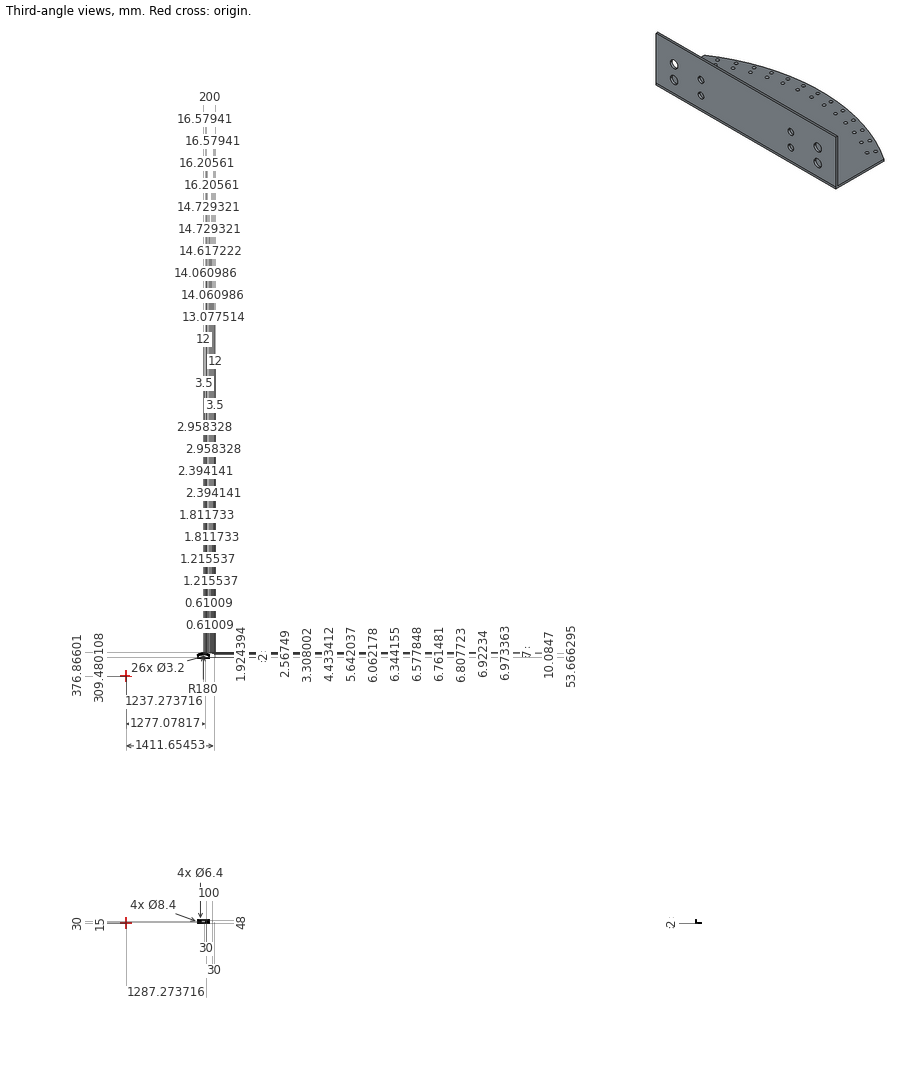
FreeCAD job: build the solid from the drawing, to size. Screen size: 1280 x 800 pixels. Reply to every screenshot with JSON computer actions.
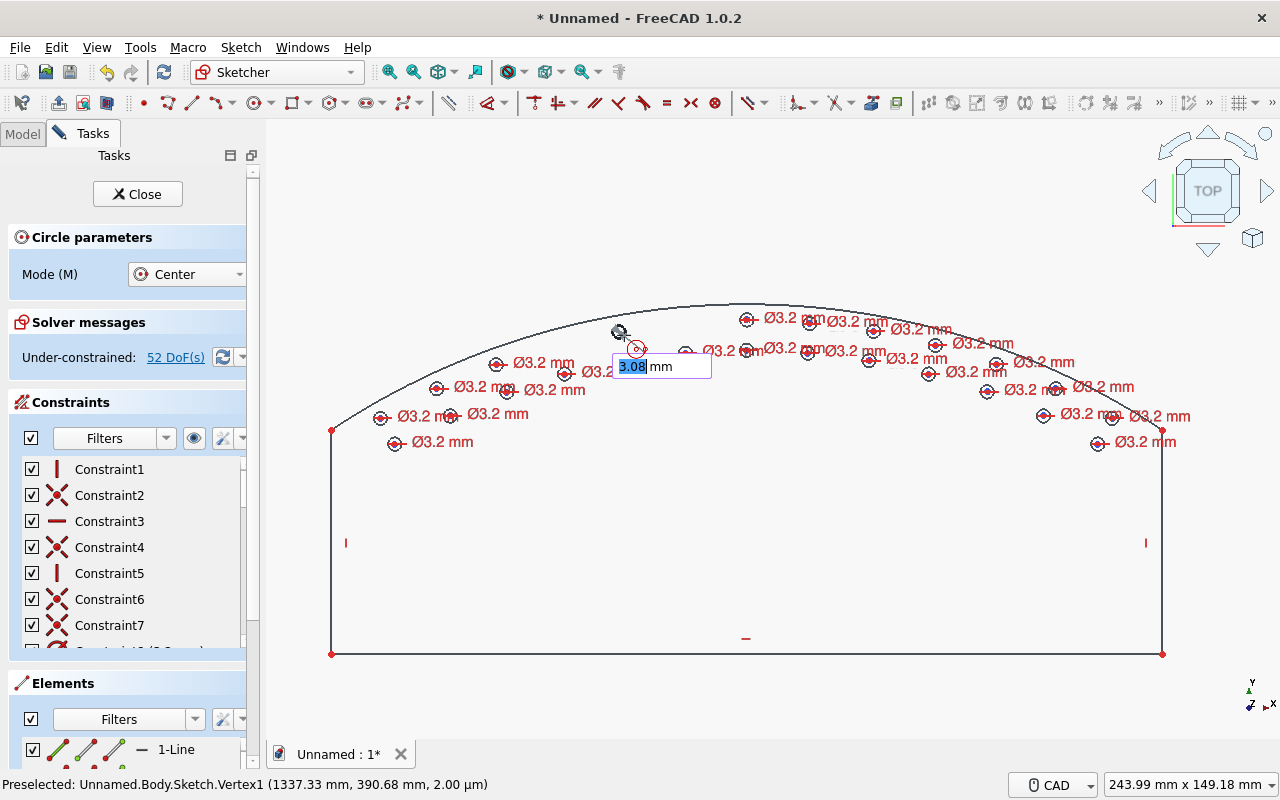
{"action": "type", "text": "3.2"}
{"action": "key", "text": "Return"}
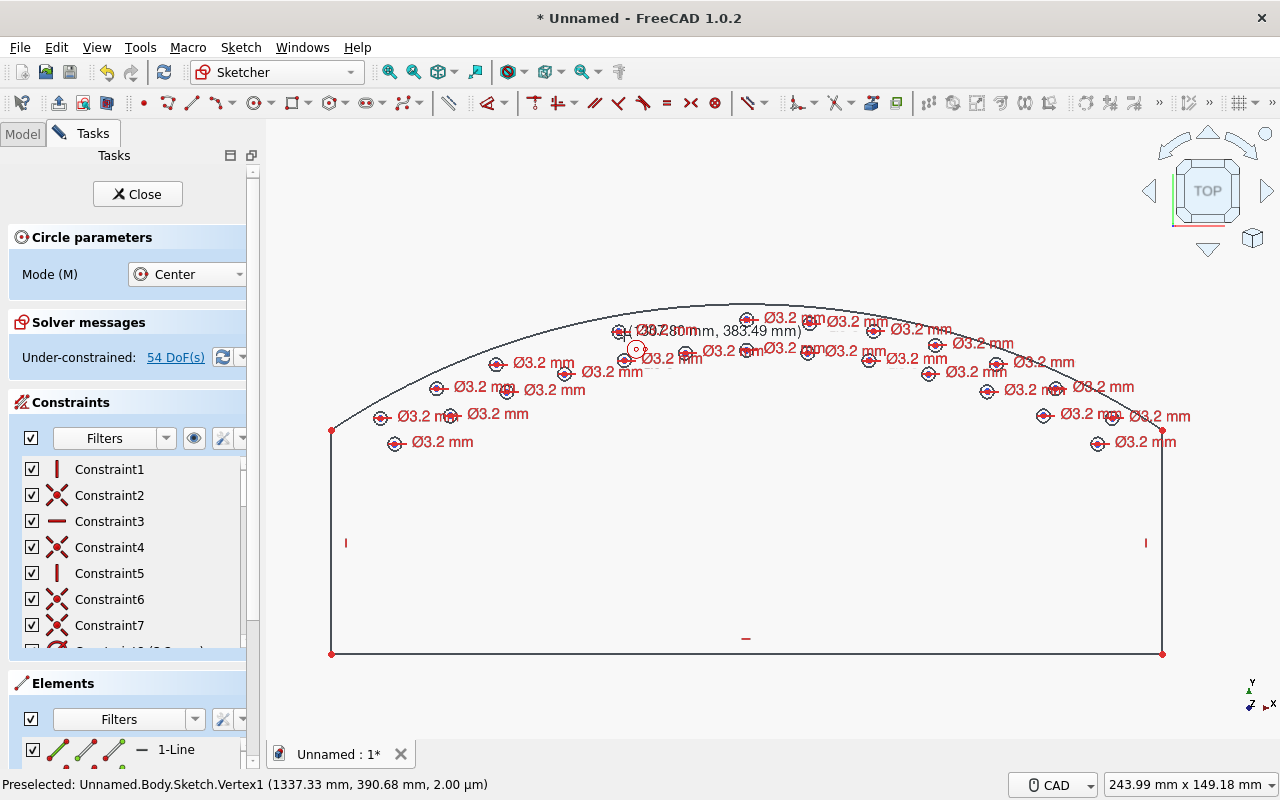
{"action": "scroll", "coordinate": [683, 322], "scroll_direction": "up", "scroll_amount": 7}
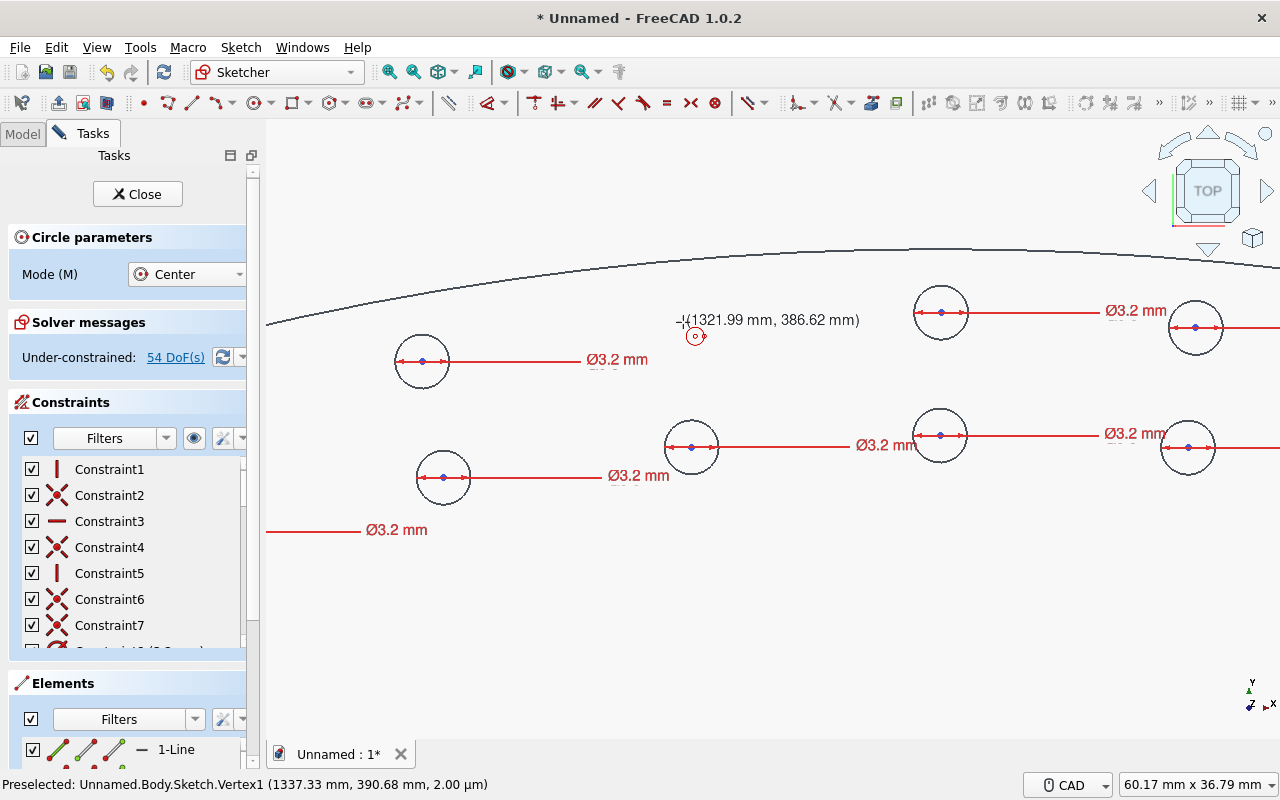
{"action": "scroll", "coordinate": [658, 326], "scroll_direction": "down", "scroll_amount": 9}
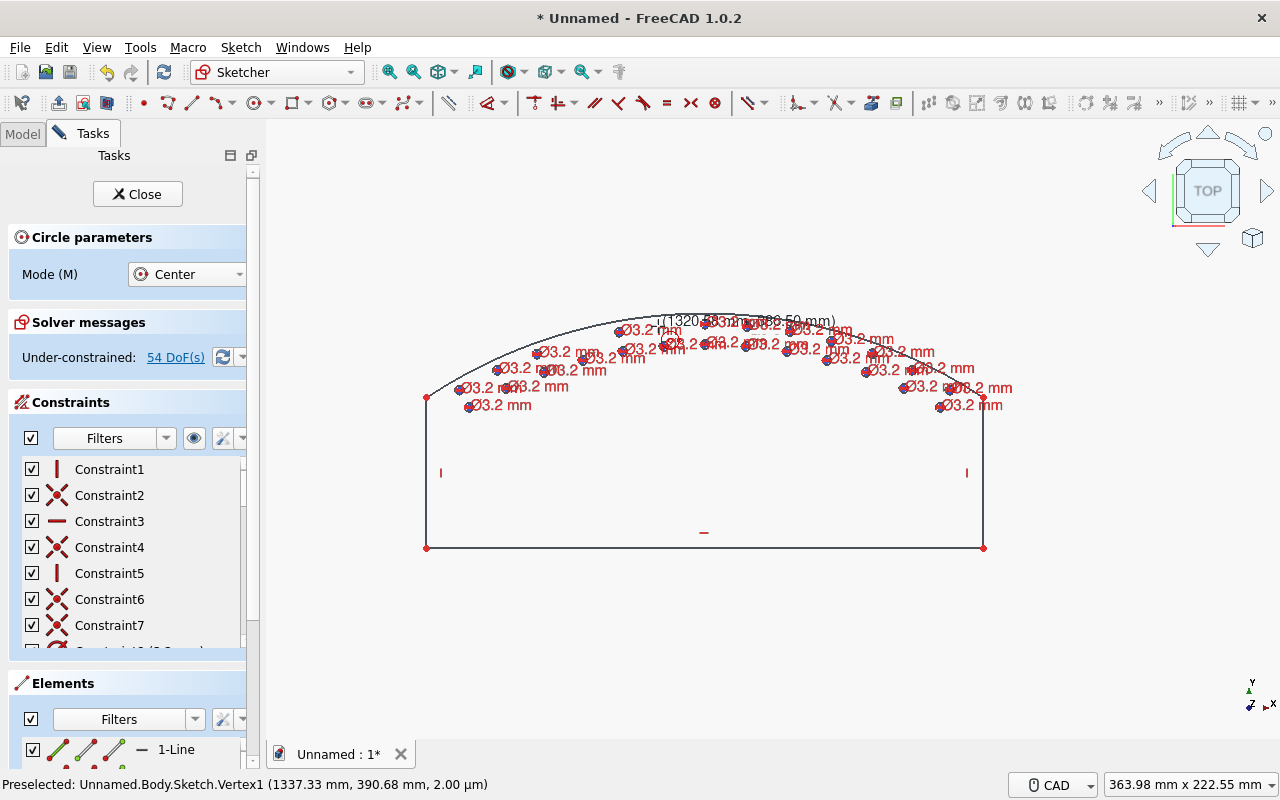
{"action": "scroll", "coordinate": [662, 326], "scroll_direction": "up", "scroll_amount": 2}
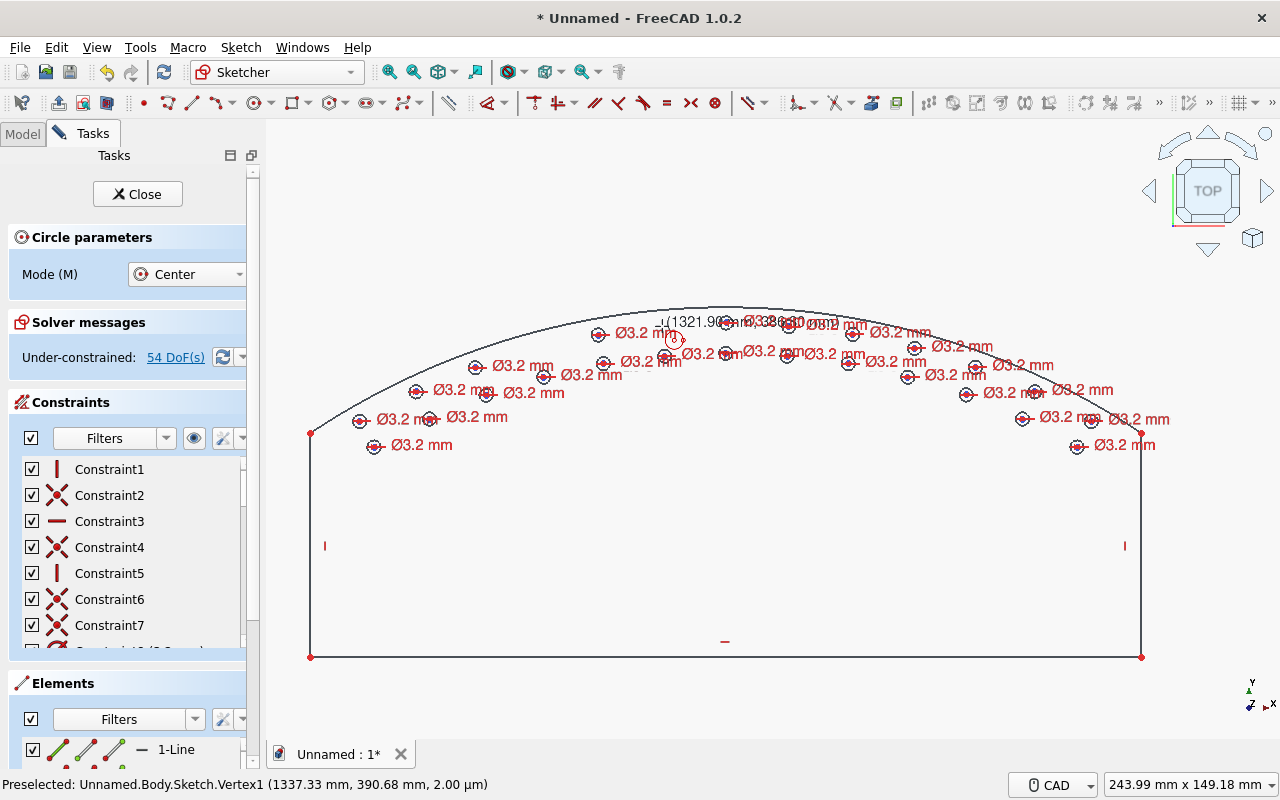
{"action": "left_click", "coordinate": [662, 325]}
{"action": "mouse_move", "coordinate": [667, 330]}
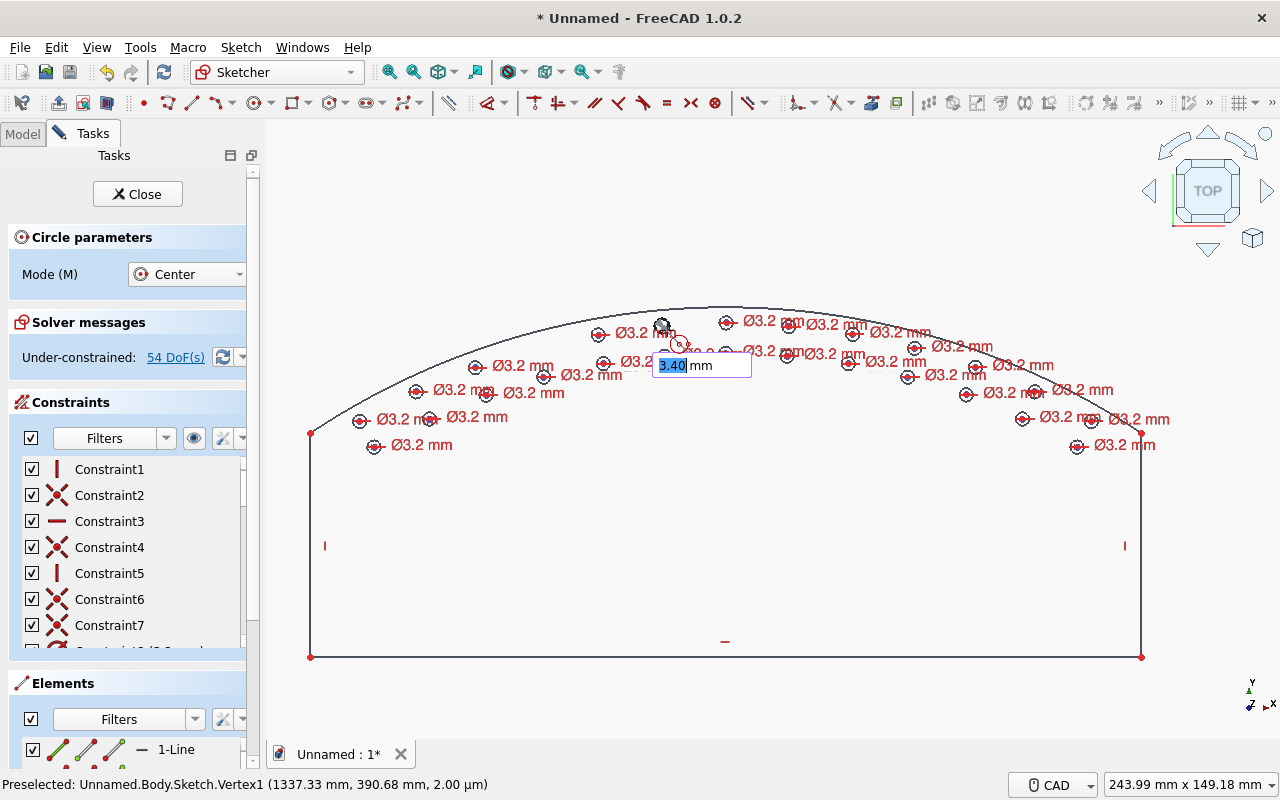
{"action": "type", "text": "3.2"}
{"action": "key", "text": "Return"}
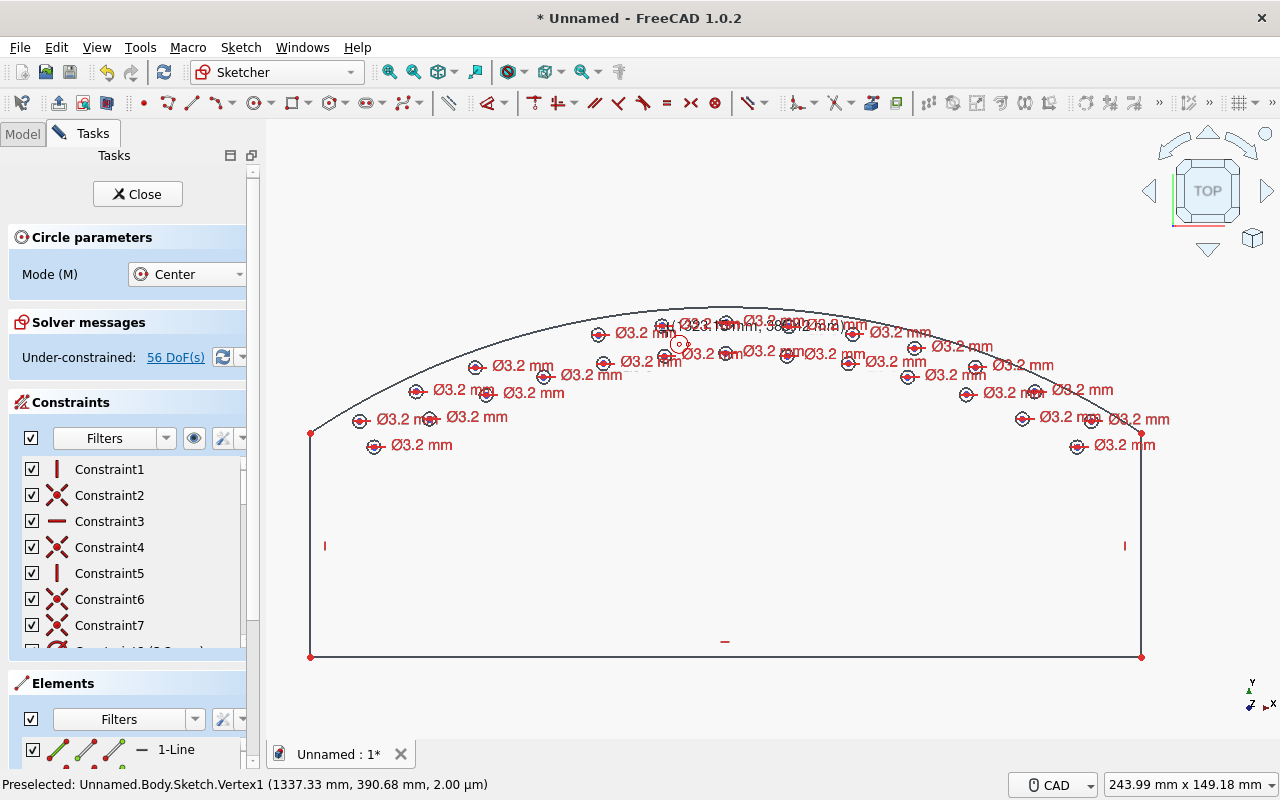
{"action": "scroll", "coordinate": [536, 347], "scroll_direction": "up", "scroll_amount": 7}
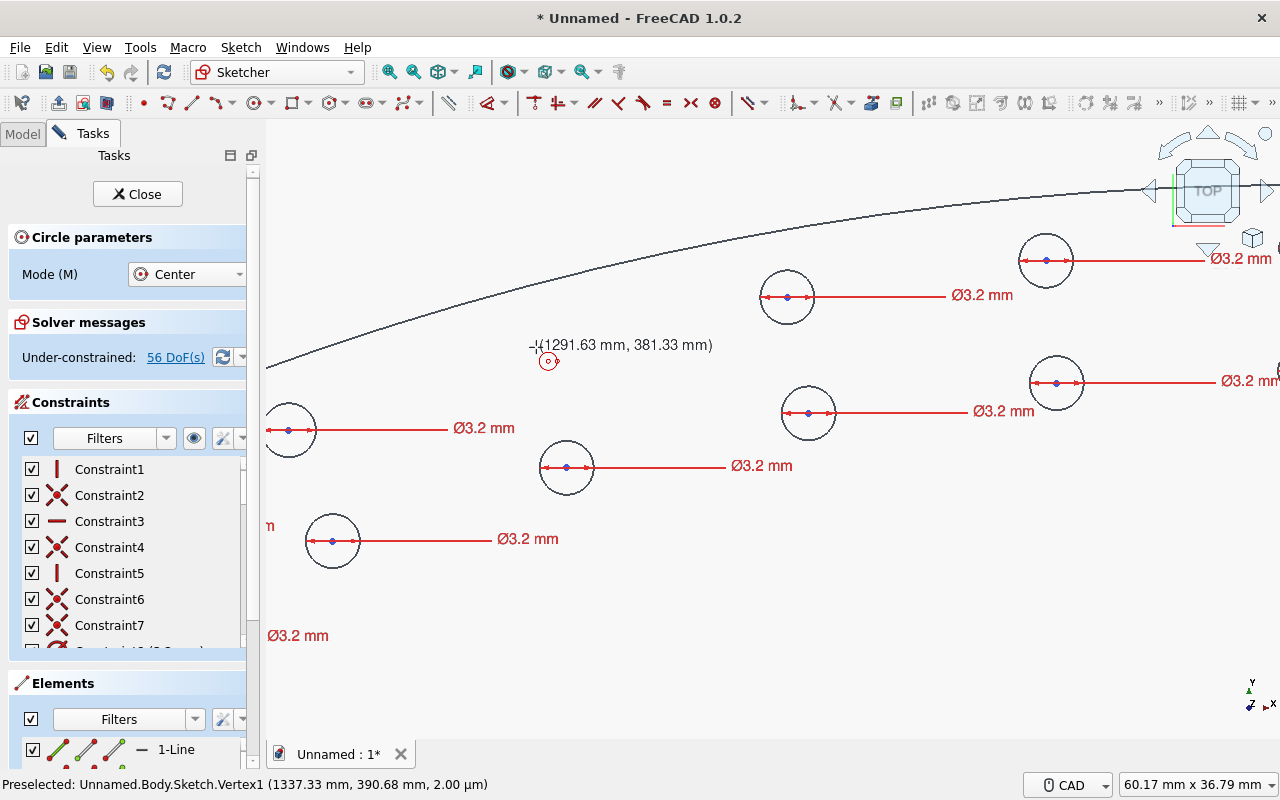
{"action": "scroll", "coordinate": [586, 338], "scroll_direction": "down", "scroll_amount": 9}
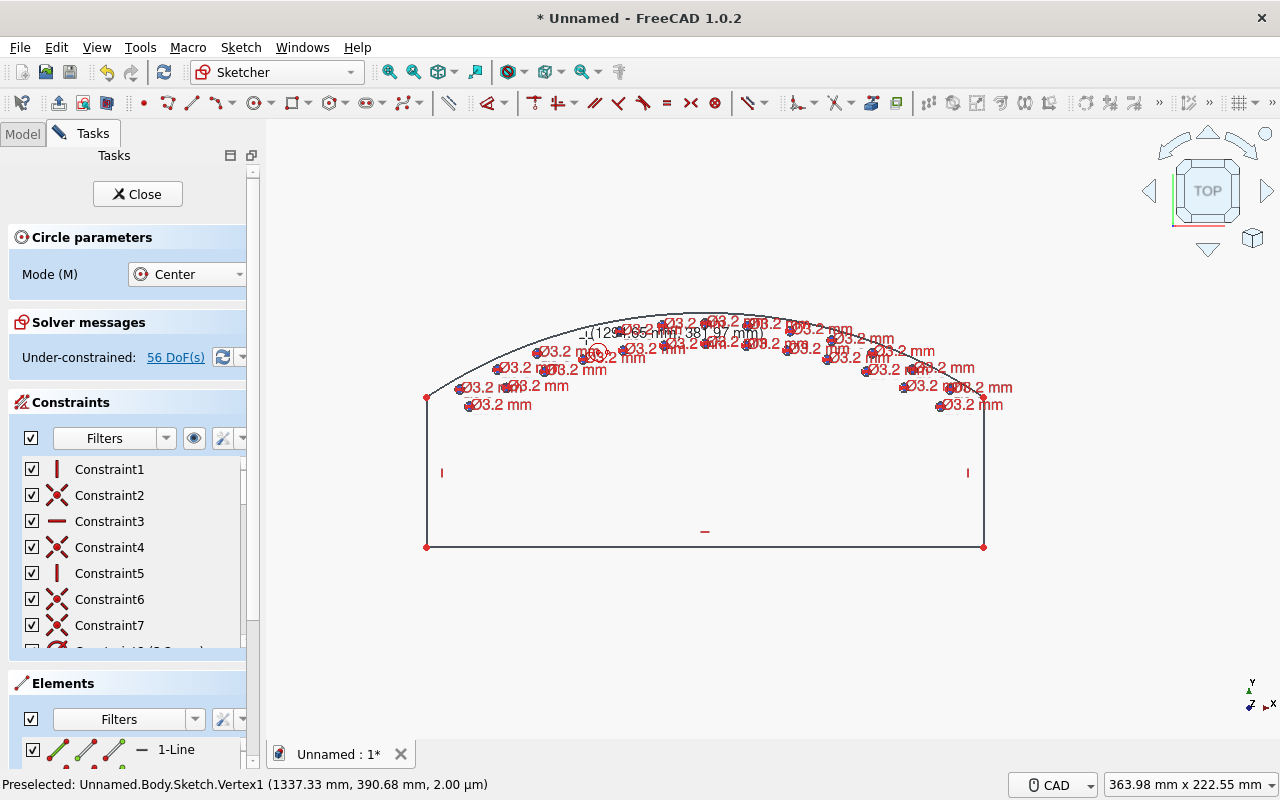
{"action": "scroll", "coordinate": [578, 340], "scroll_direction": "up", "scroll_amount": 2}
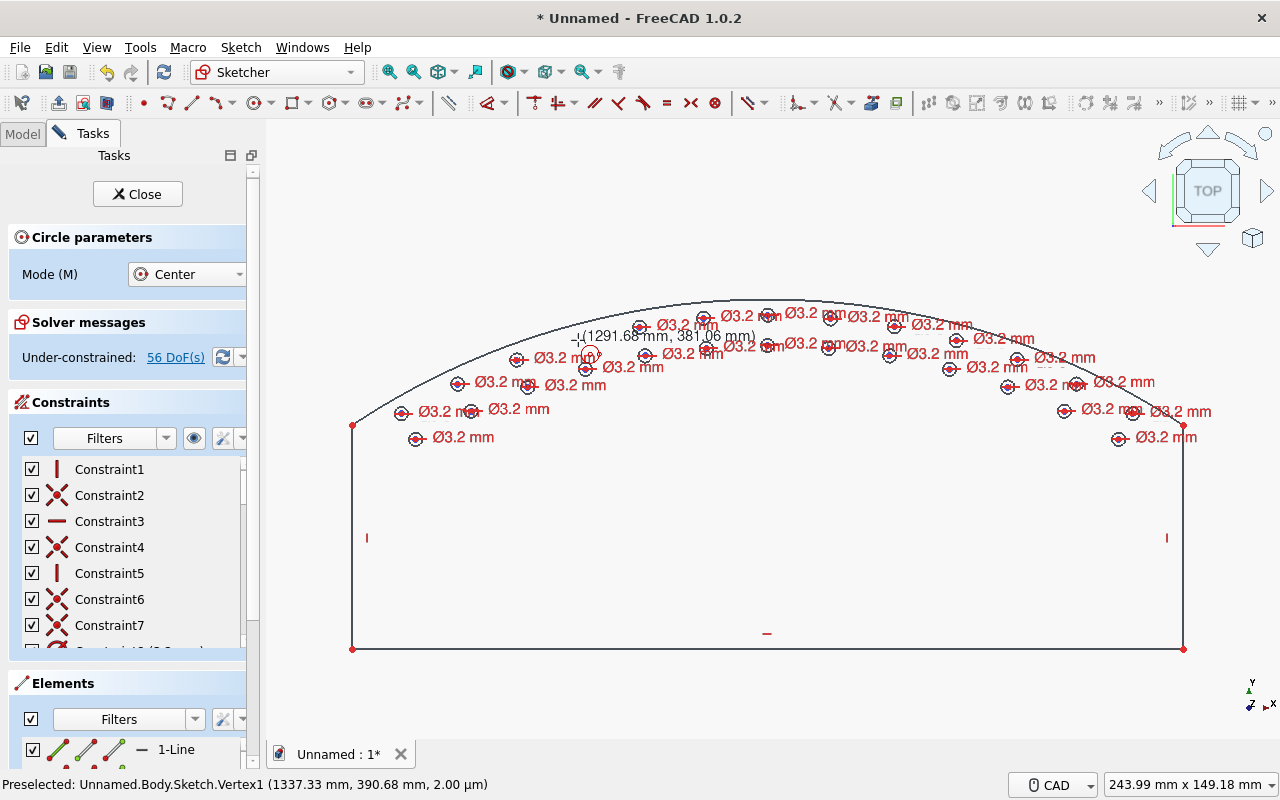
{"action": "left_click", "coordinate": [578, 340]}
{"action": "mouse_move", "coordinate": [583, 344]}